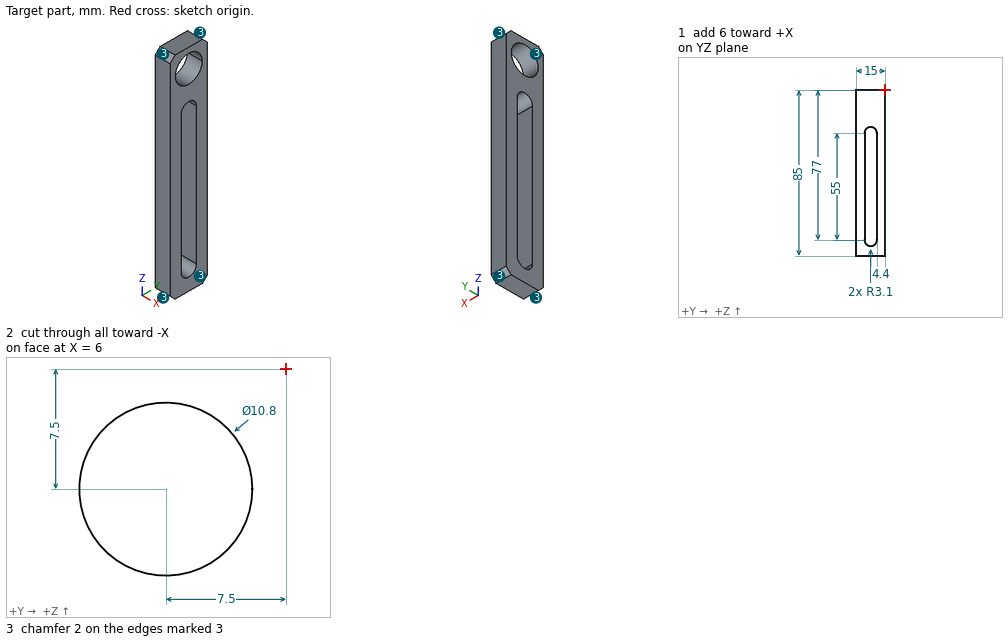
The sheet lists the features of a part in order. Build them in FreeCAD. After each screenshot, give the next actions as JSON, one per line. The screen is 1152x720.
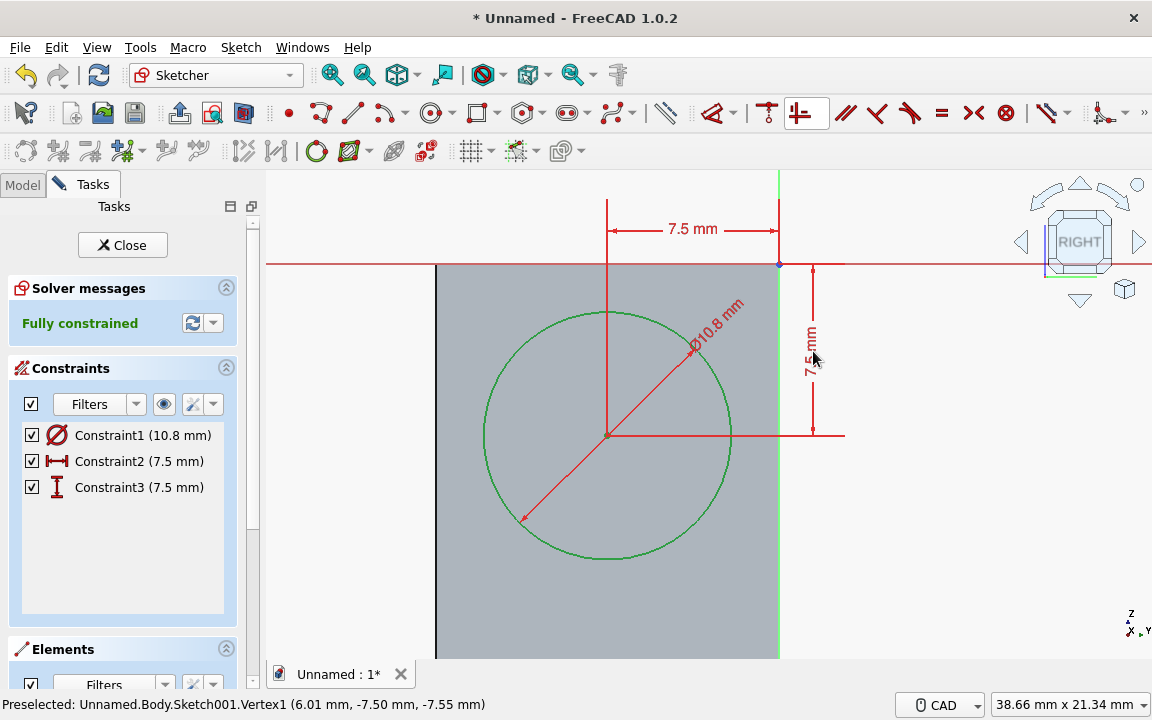
{"action": "left_click", "coordinate": [123, 245]}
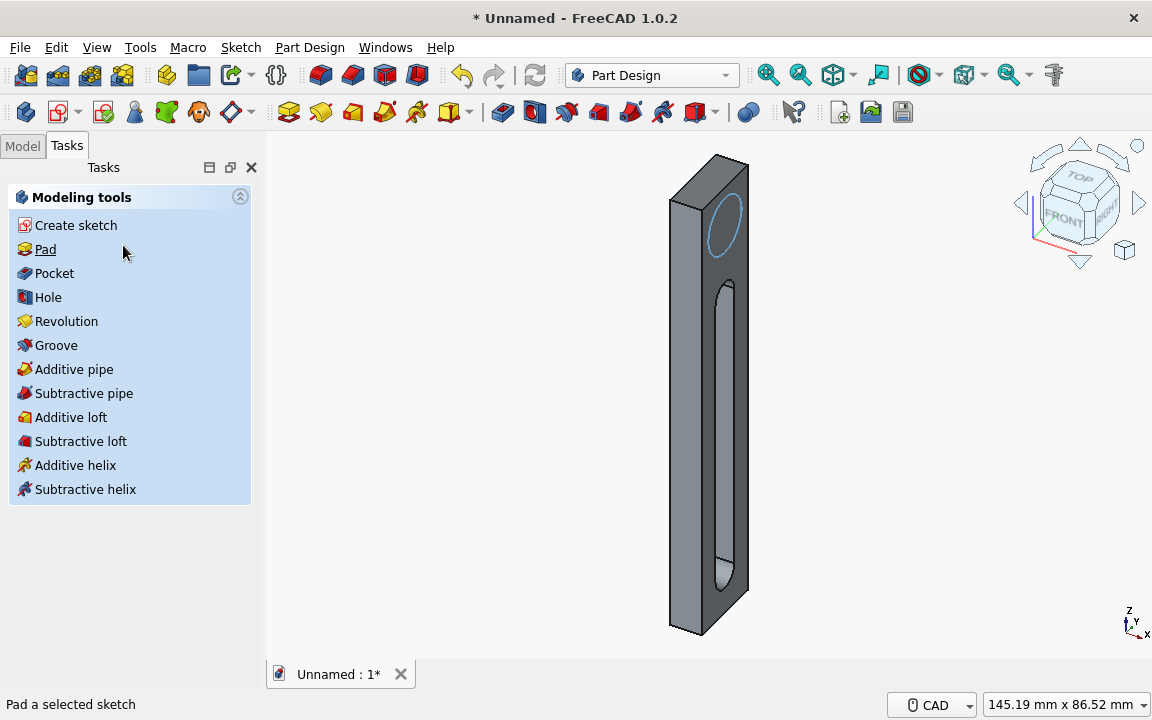
{"action": "left_click", "coordinate": [504, 112]}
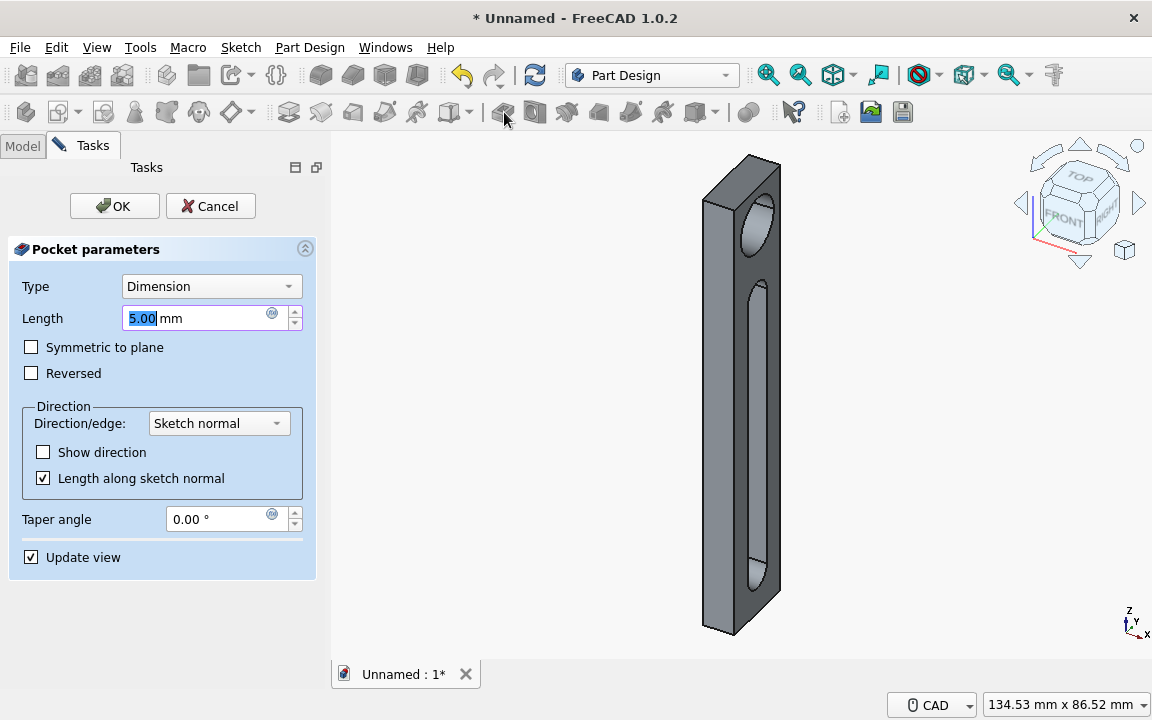
{"action": "left_click", "coordinate": [212, 286]}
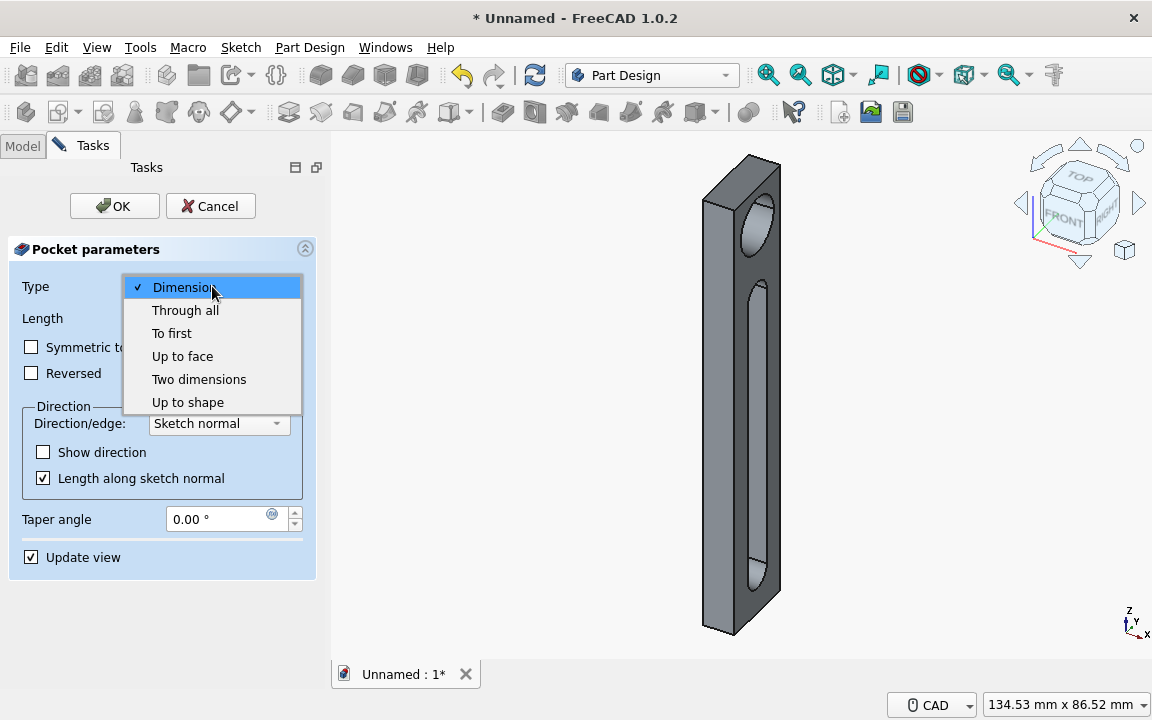
{"action": "left_click", "coordinate": [212, 310]}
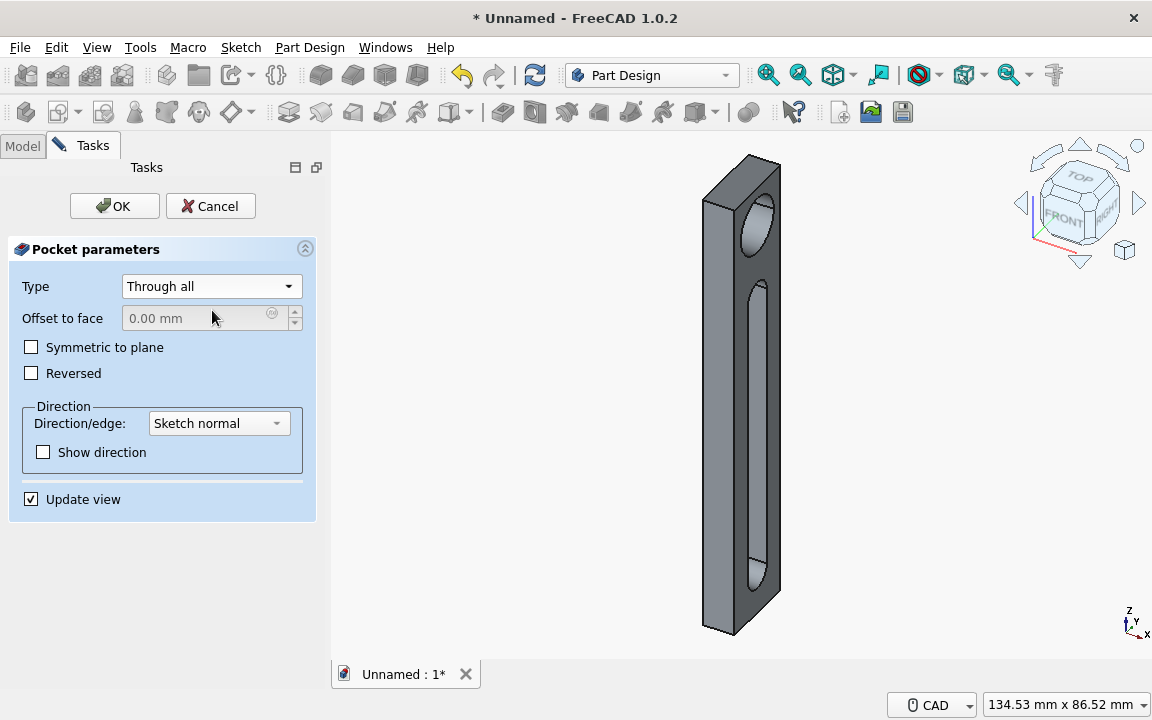
{"action": "left_click", "coordinate": [115, 206]}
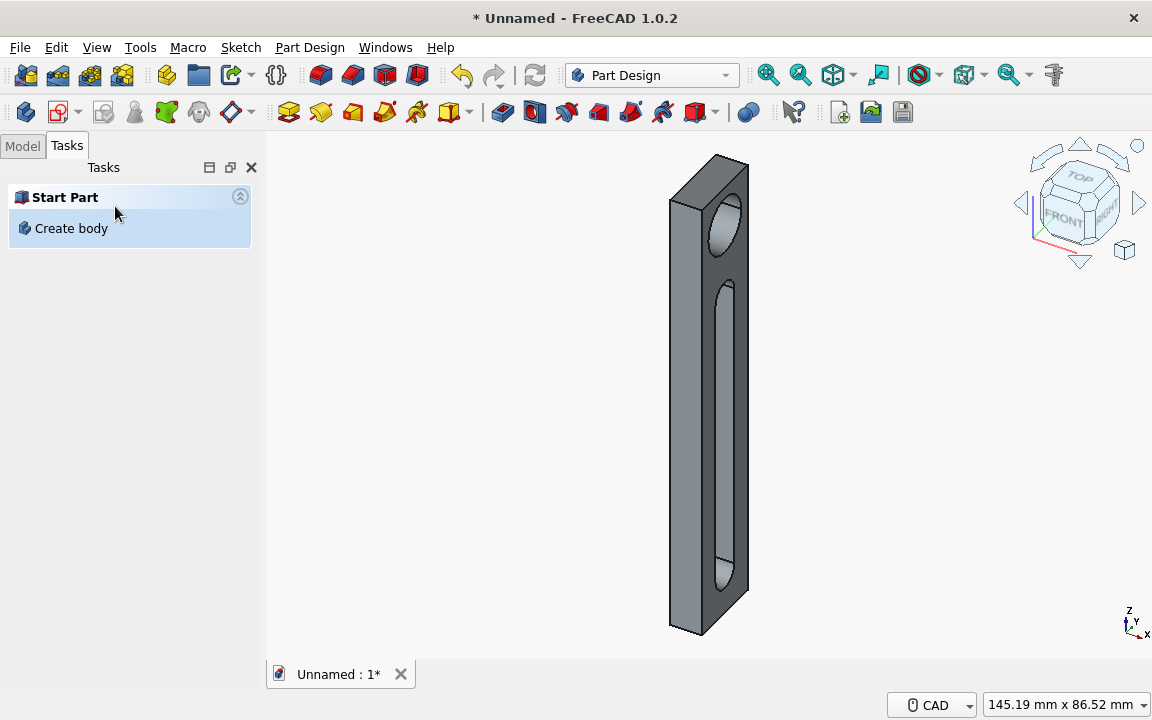
{"action": "left_click", "coordinate": [686, 204]}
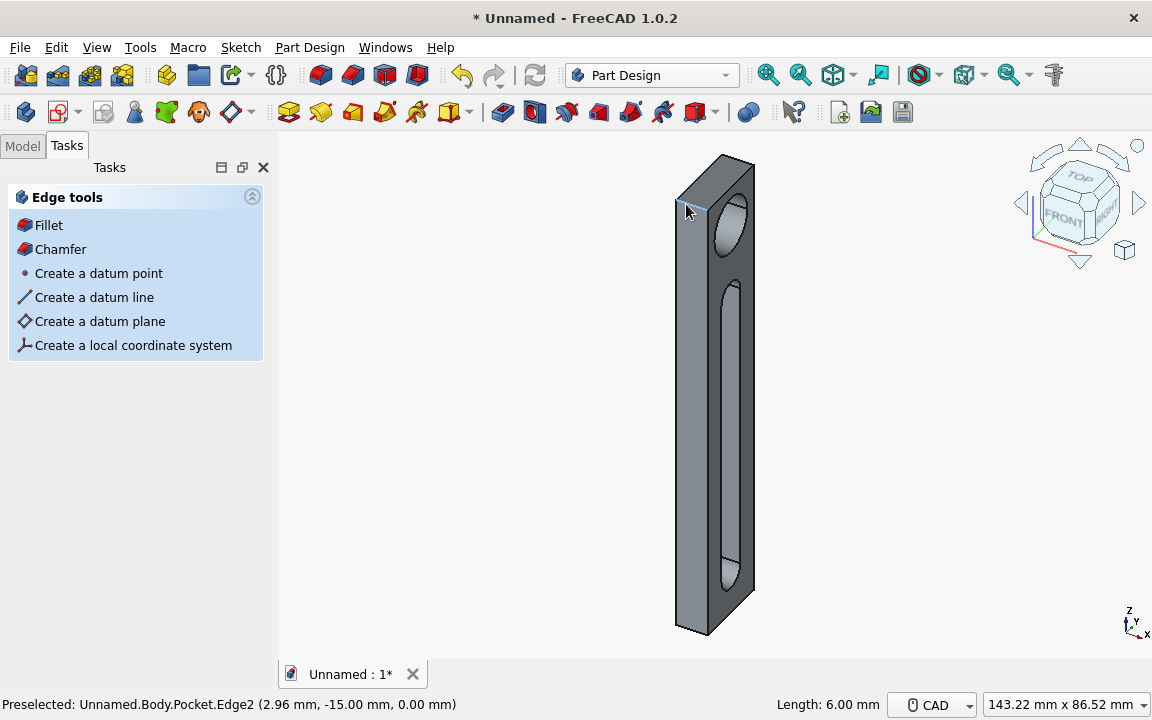
{"action": "key", "text": "0"}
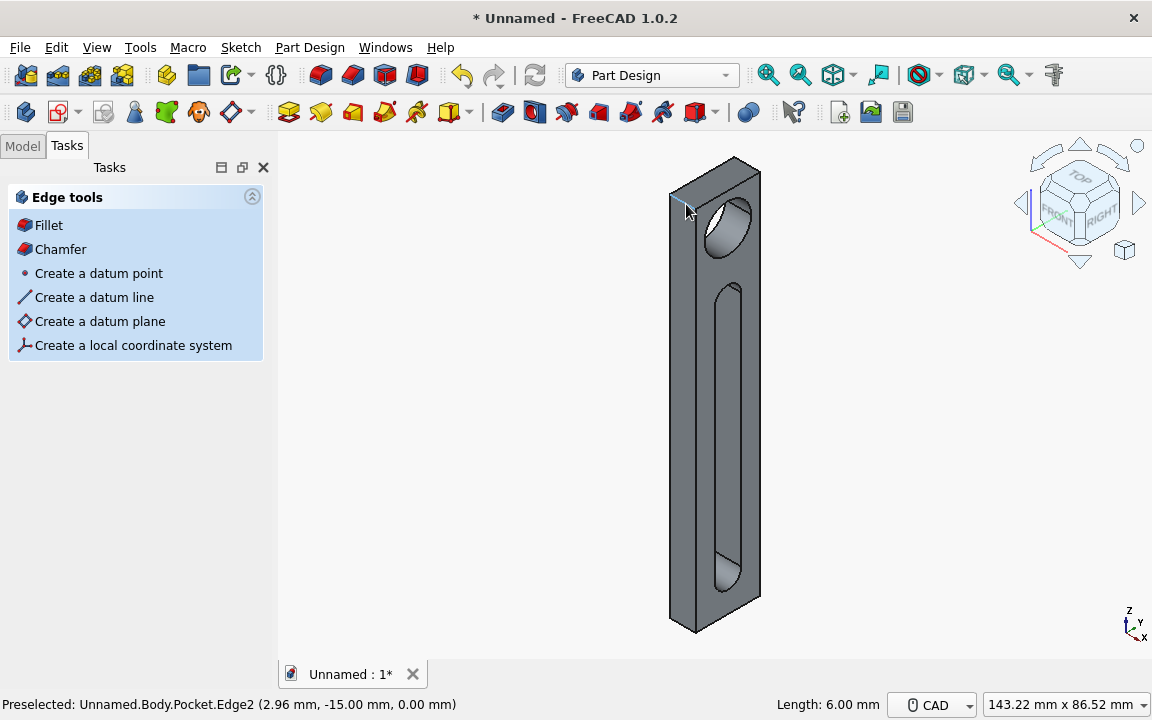
{"action": "key", "text": "2"}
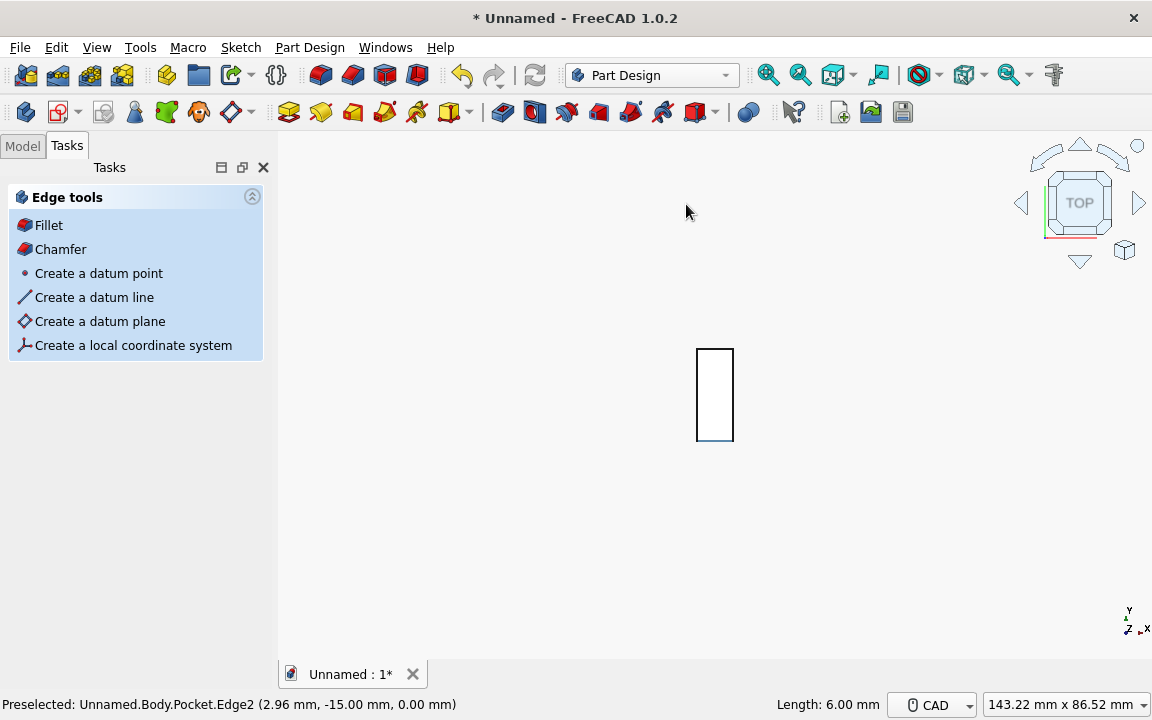
{"action": "left_click", "coordinate": [770, 76]}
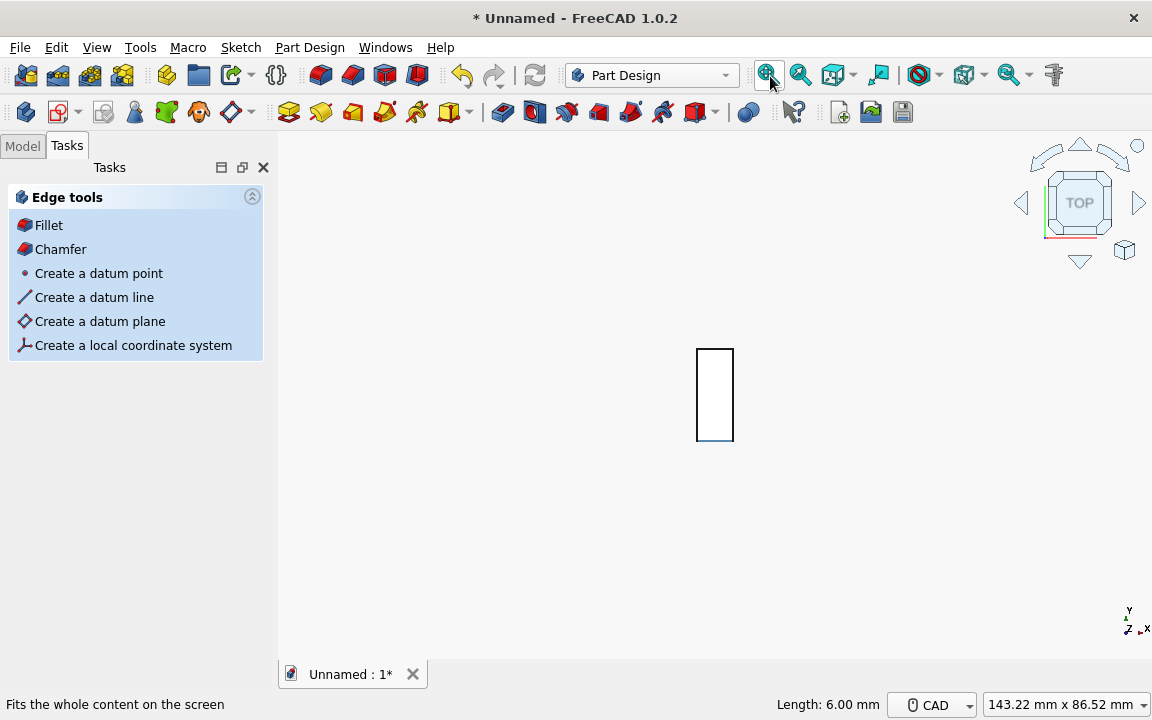
{"action": "key", "text": "1"}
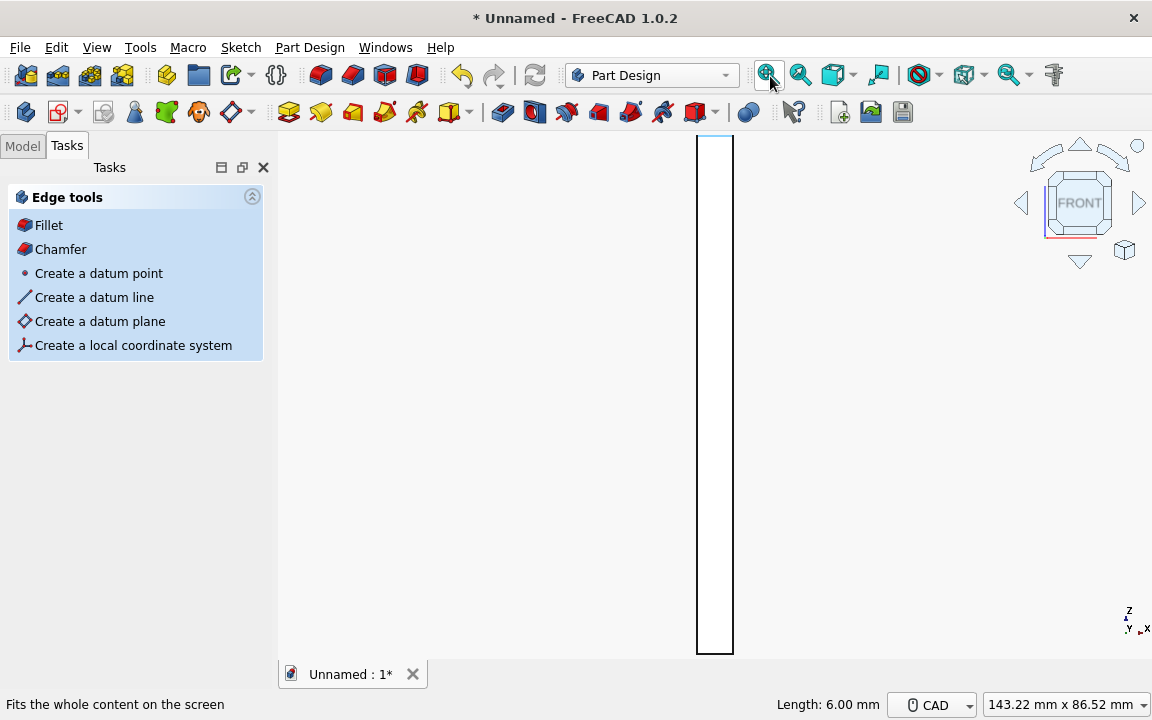
{"action": "key", "text": "3"}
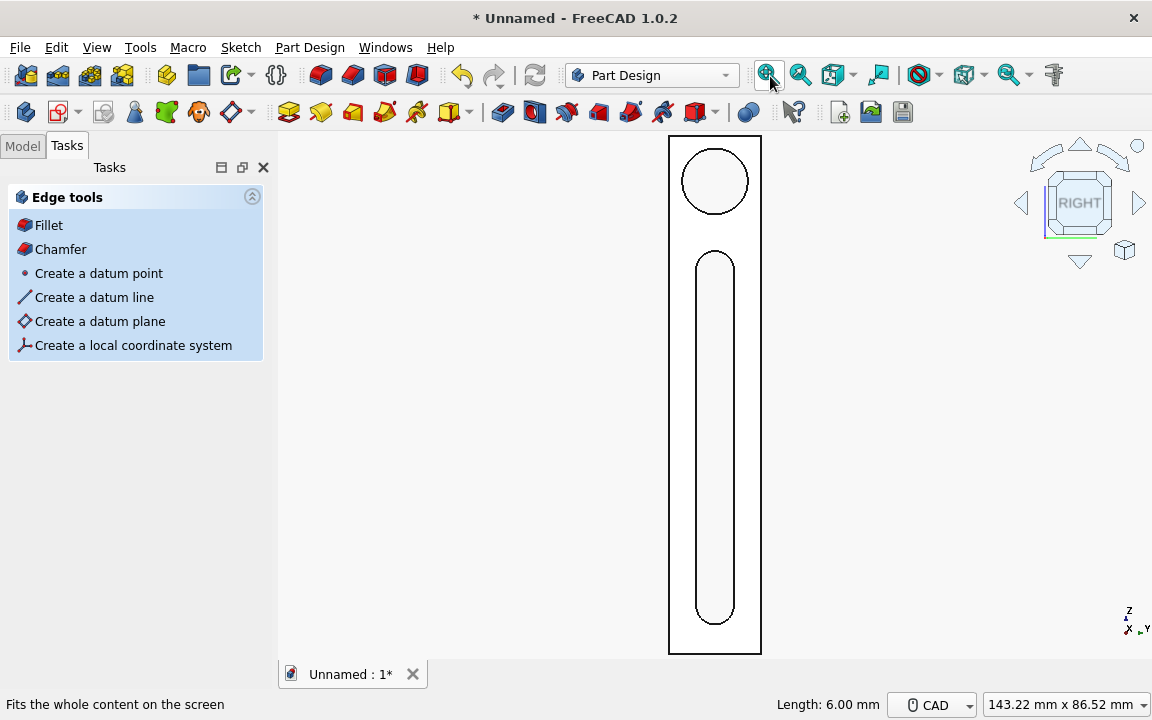
{"action": "key", "text": "5"}